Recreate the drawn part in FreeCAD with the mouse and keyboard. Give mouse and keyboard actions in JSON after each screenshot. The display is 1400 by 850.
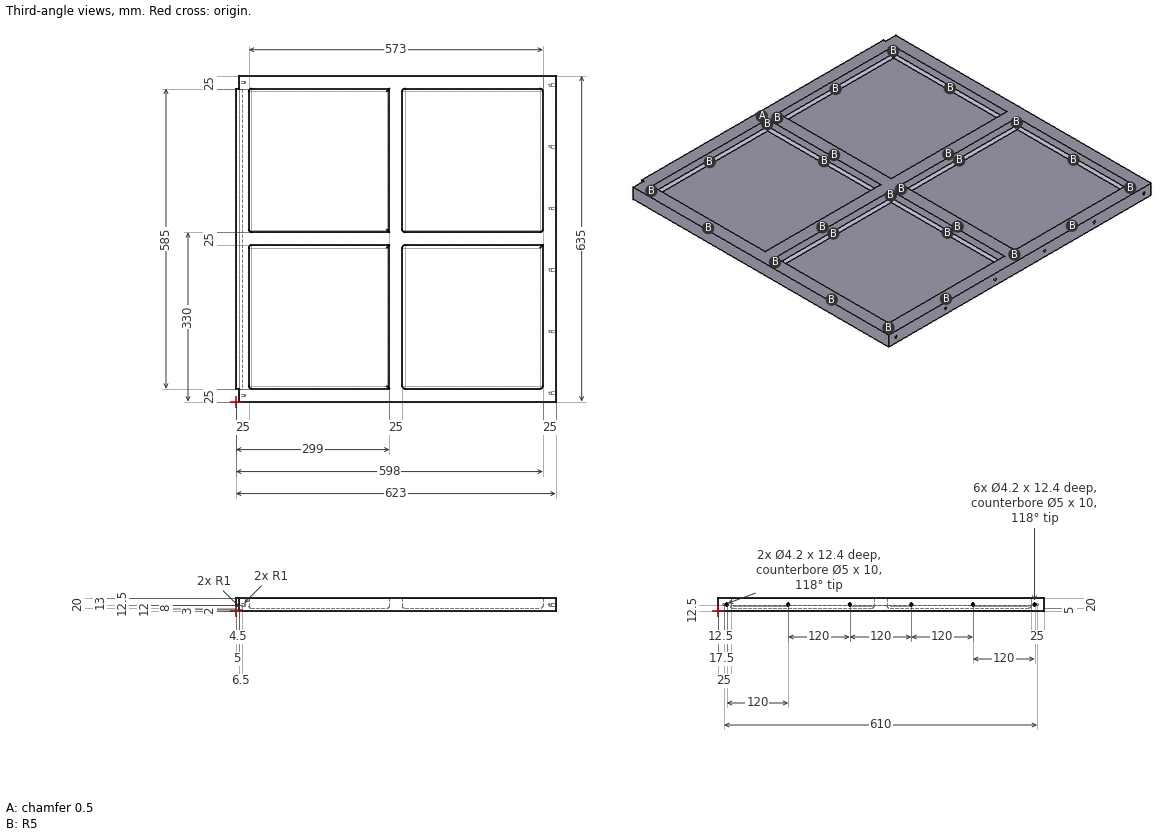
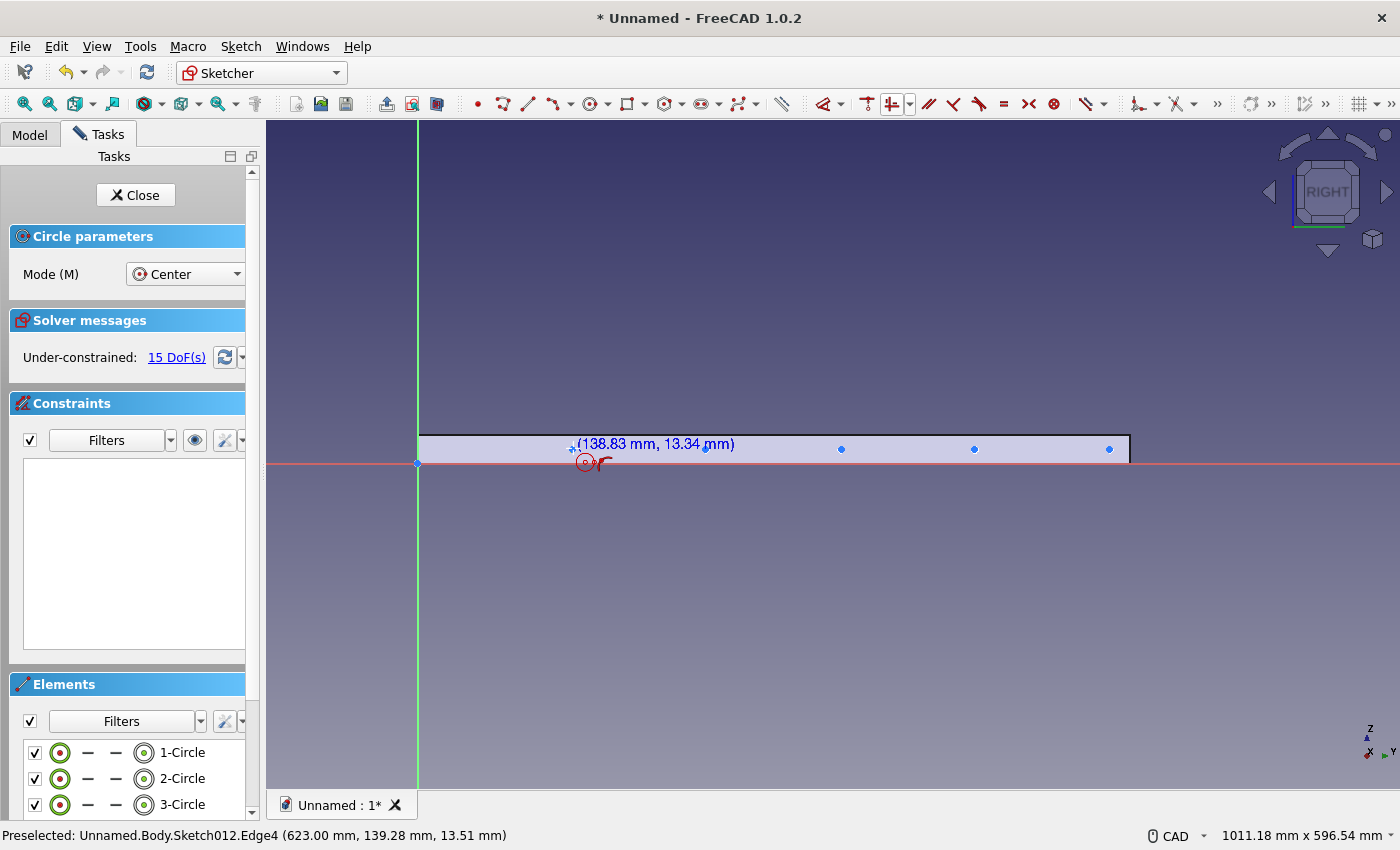
{"action": "scroll", "coordinate": [437, 449], "scroll_direction": "up", "scroll_amount": 12}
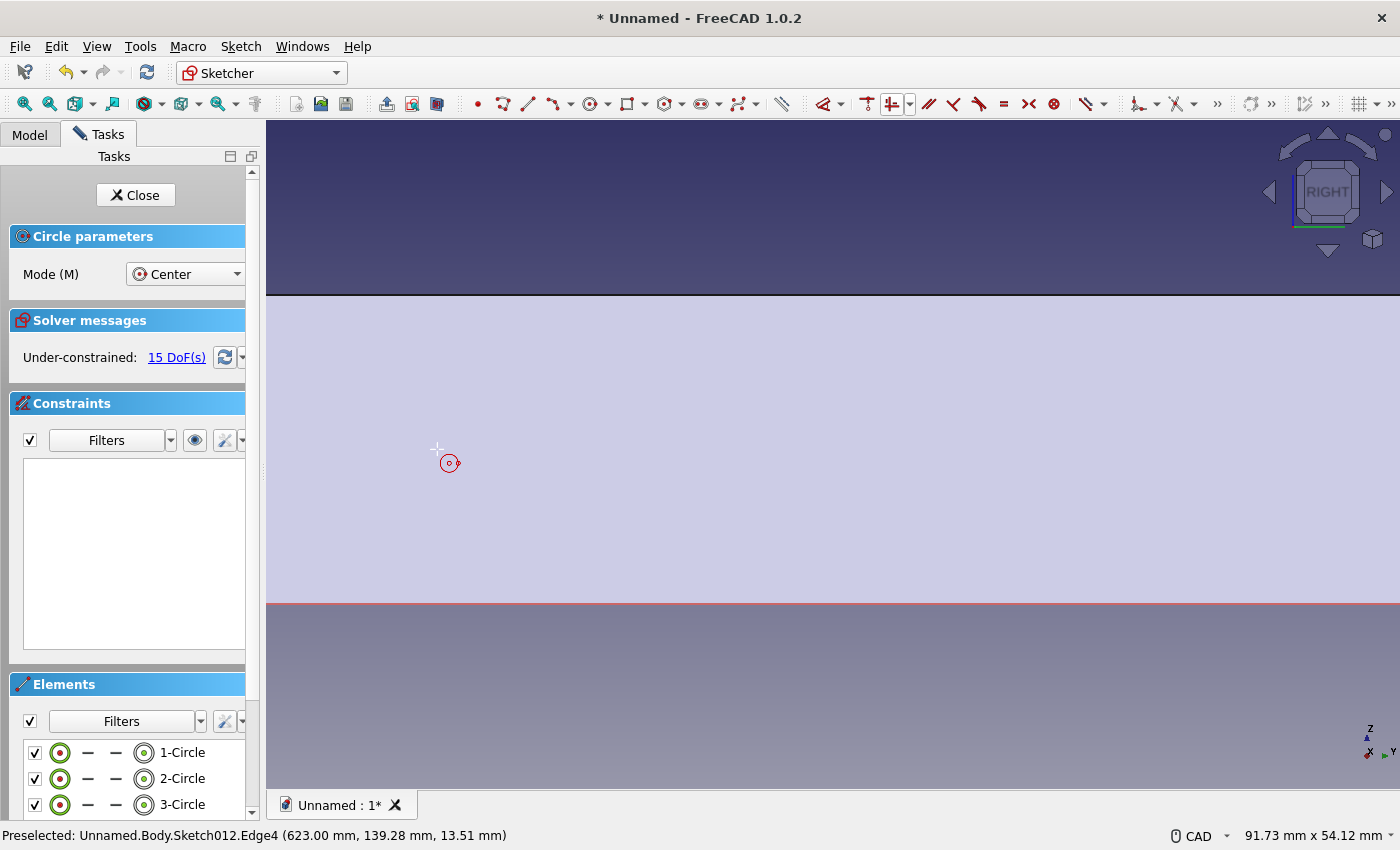
{"action": "scroll", "coordinate": [437, 449], "scroll_direction": "down", "scroll_amount": 12}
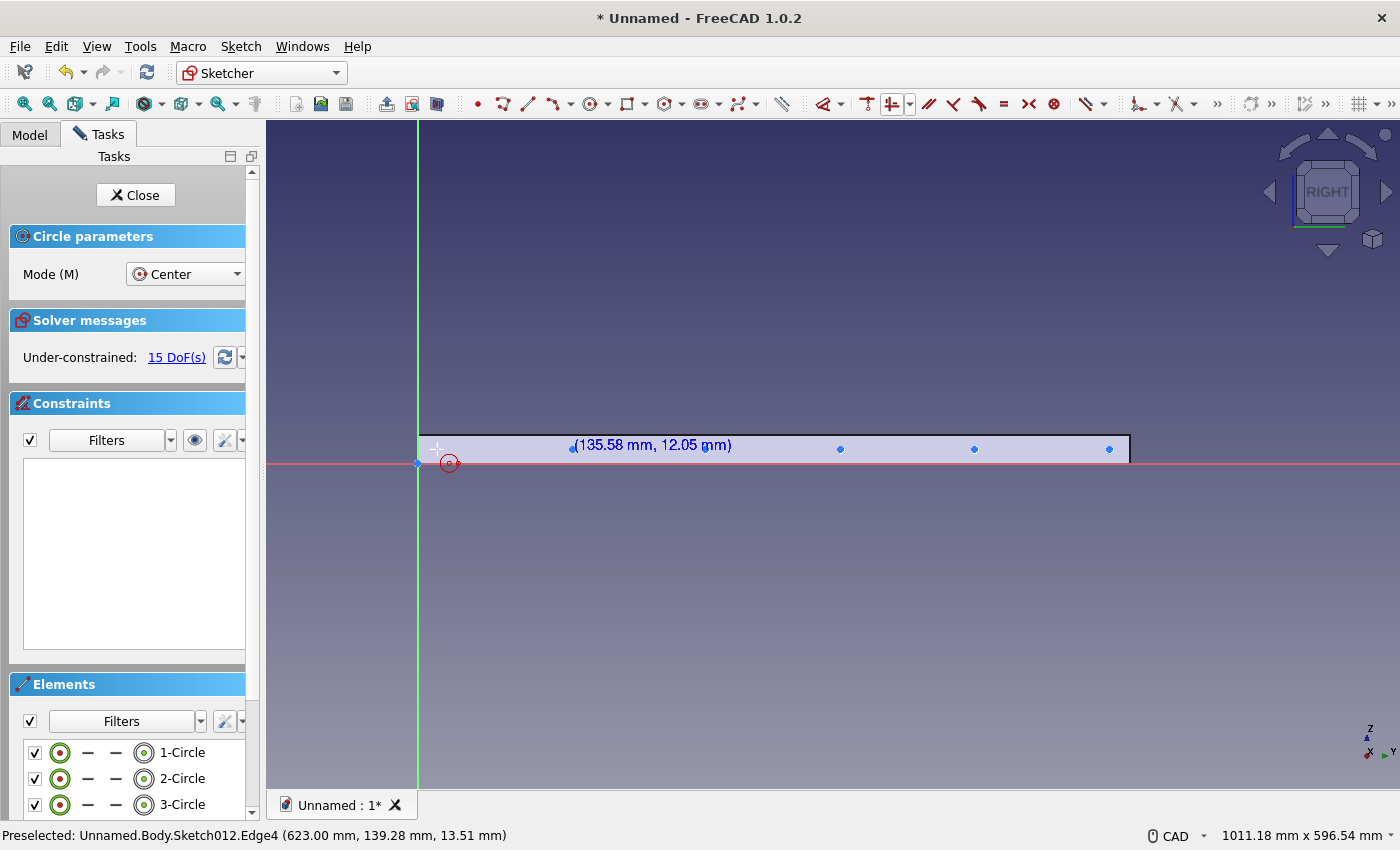
{"action": "left_click", "coordinate": [437, 449]}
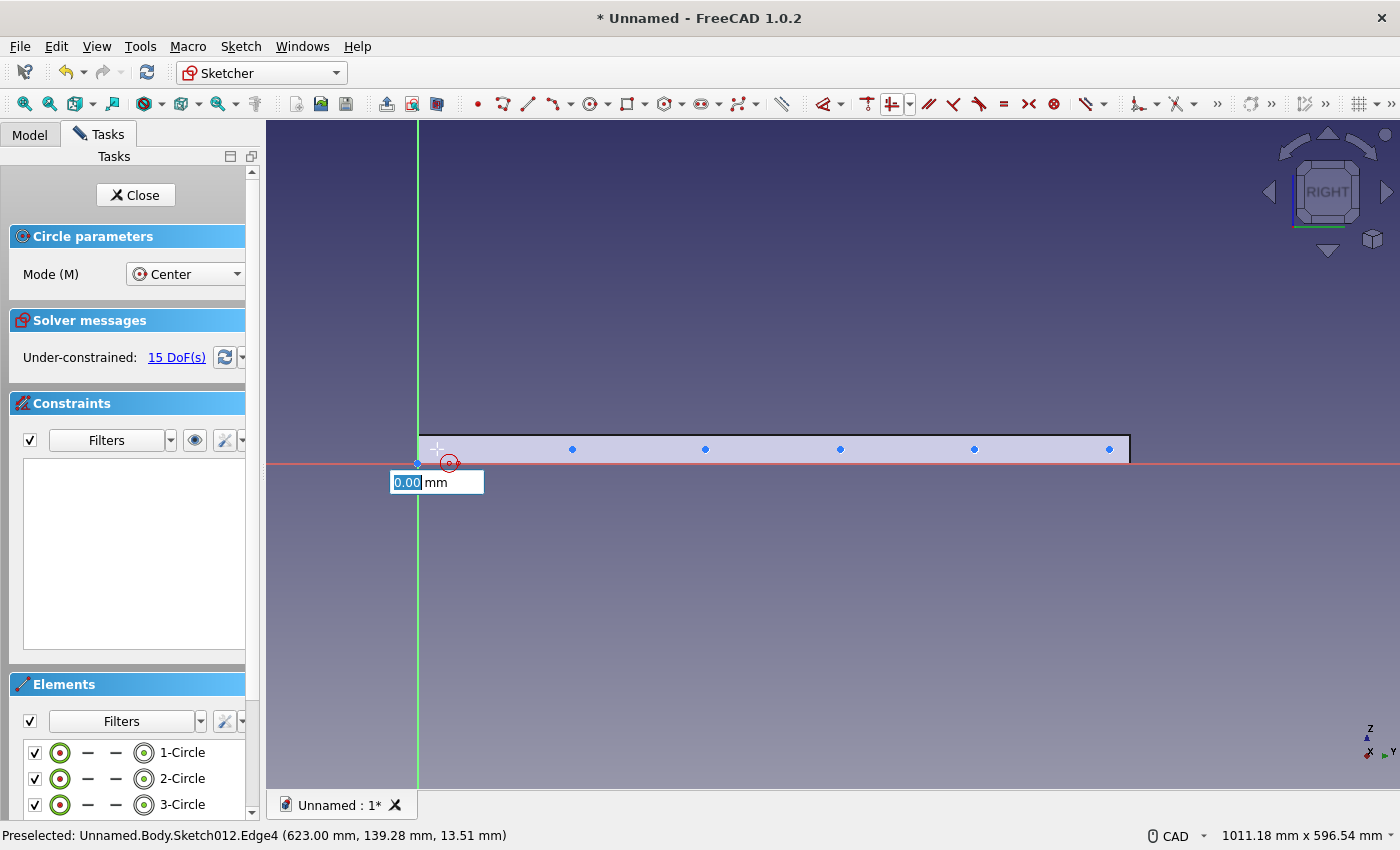
{"action": "scroll", "coordinate": [439, 448], "scroll_direction": "up", "scroll_amount": 10}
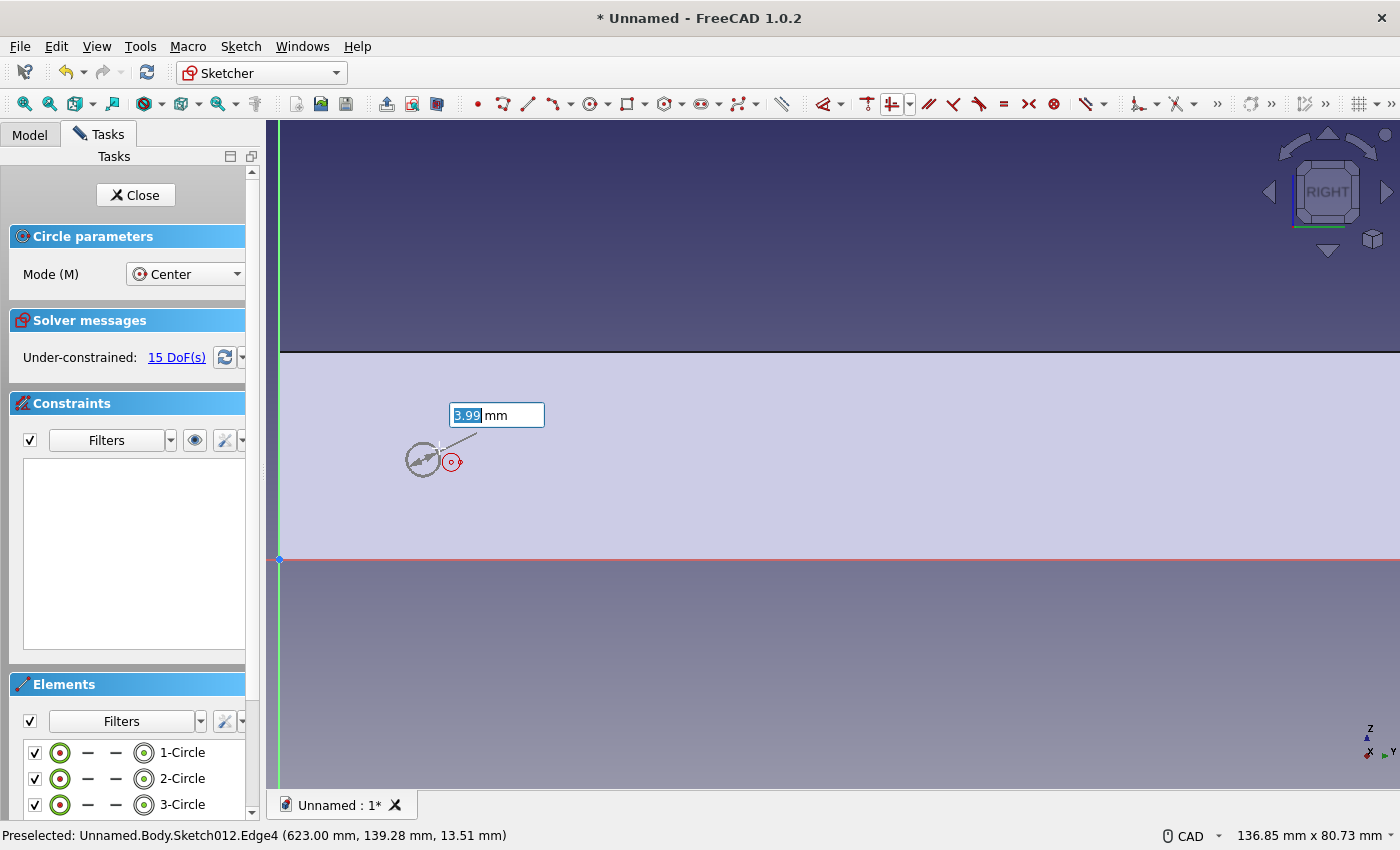
{"action": "left_click", "coordinate": [437, 444]}
{"action": "key", "text": "Escape"}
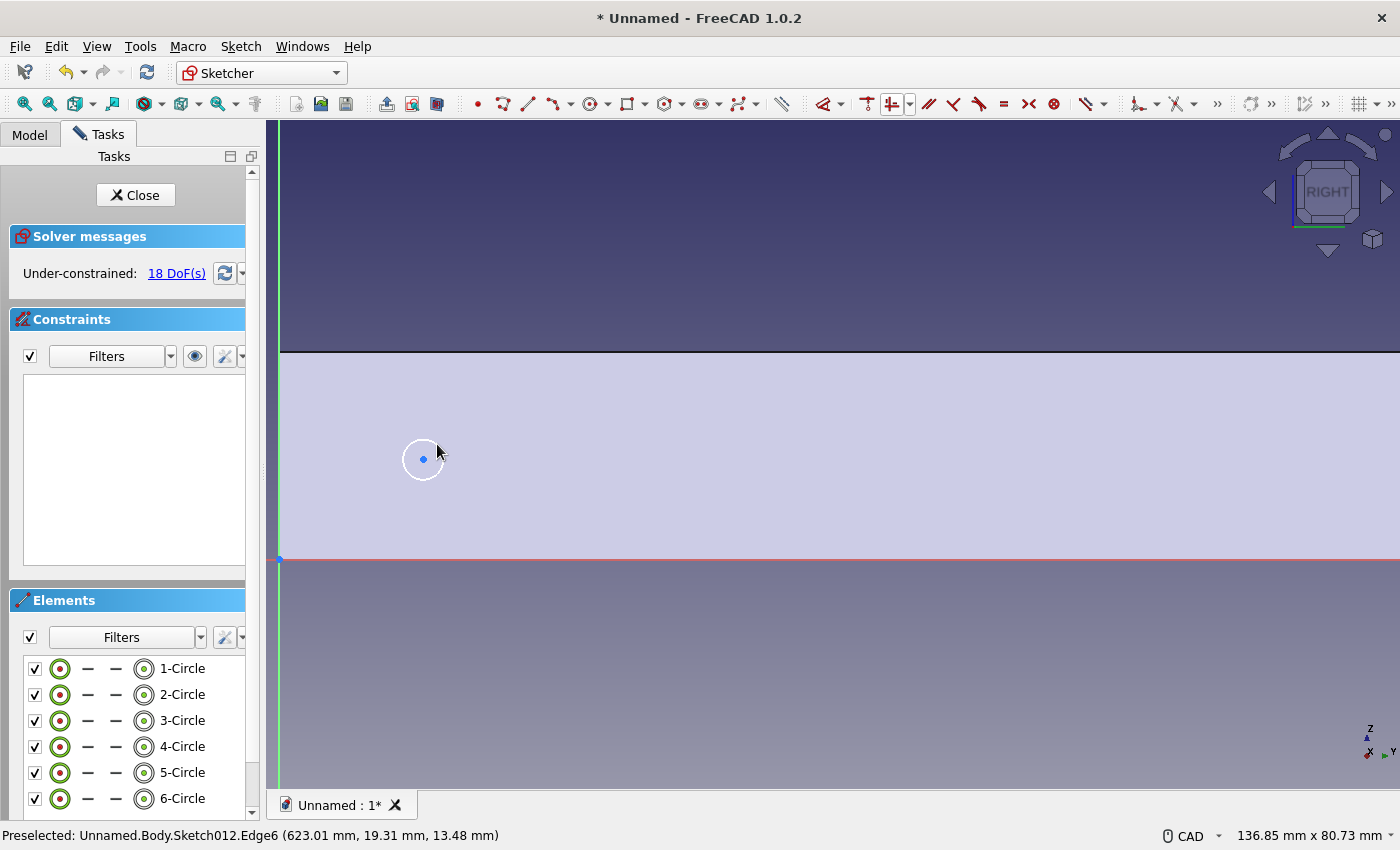
{"action": "scroll", "coordinate": [439, 448], "scroll_direction": "down", "scroll_amount": 10}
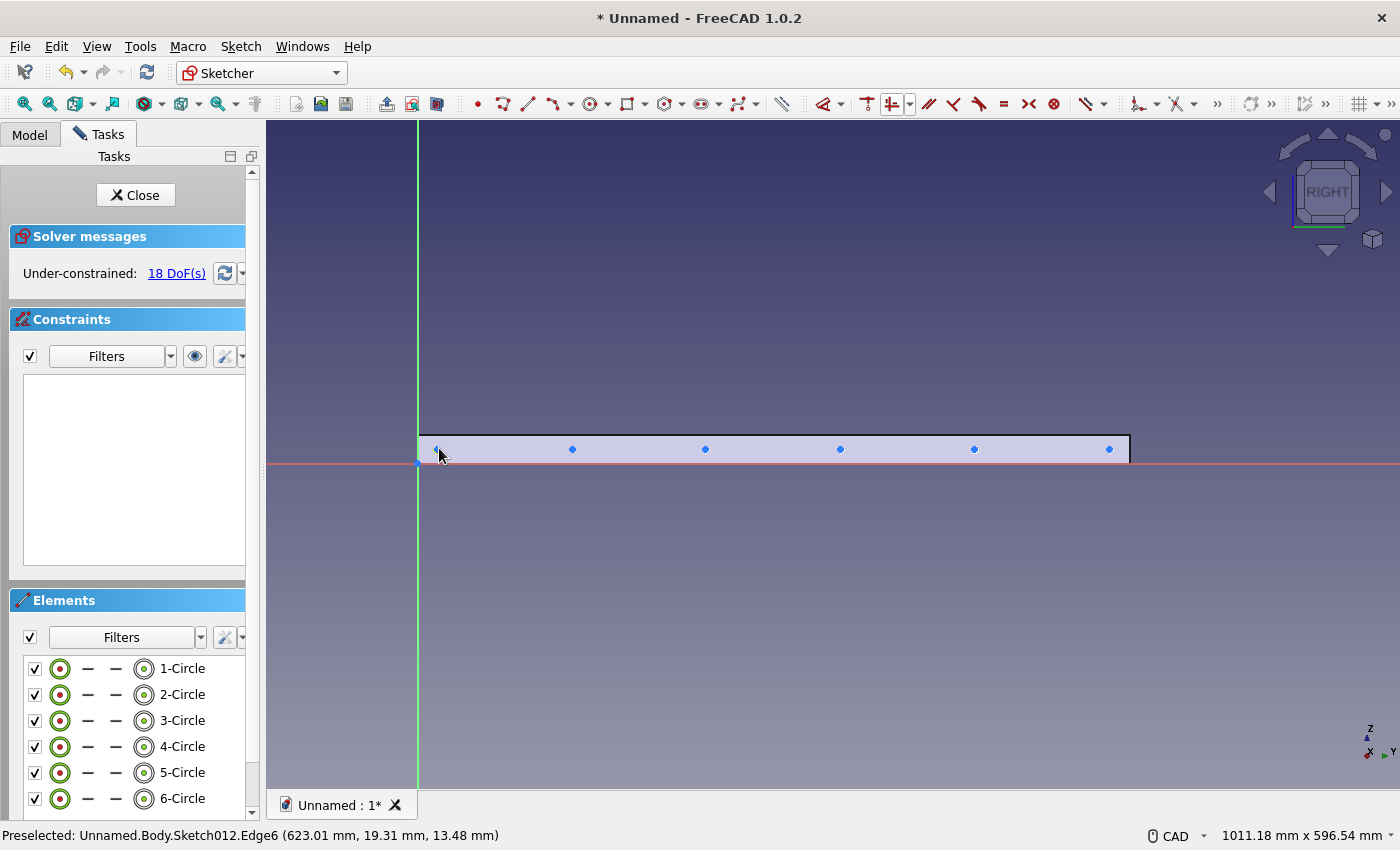
{"action": "scroll", "coordinate": [1112, 448], "scroll_direction": "up", "scroll_amount": 9}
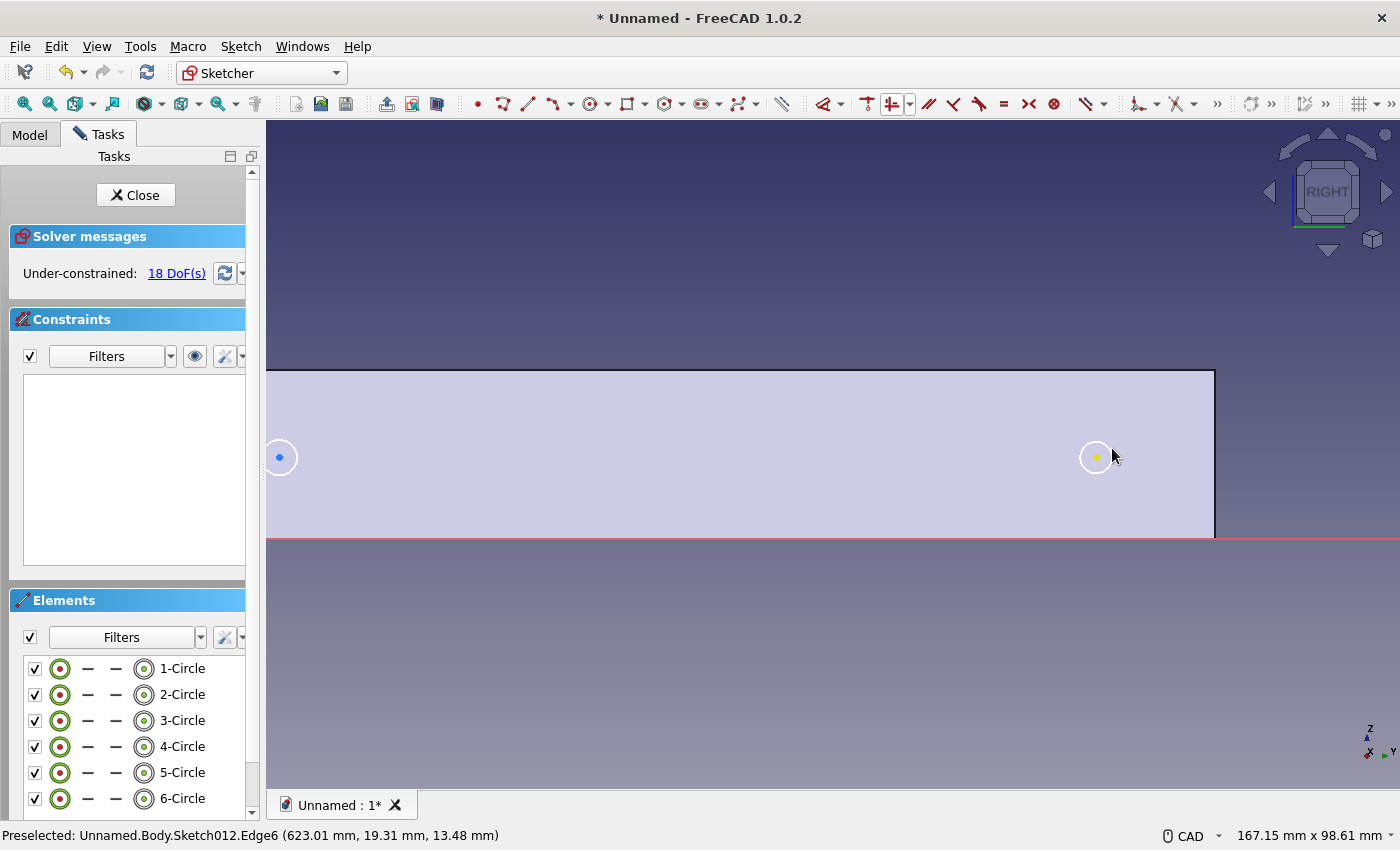
{"action": "left_click", "coordinate": [1107, 446]}